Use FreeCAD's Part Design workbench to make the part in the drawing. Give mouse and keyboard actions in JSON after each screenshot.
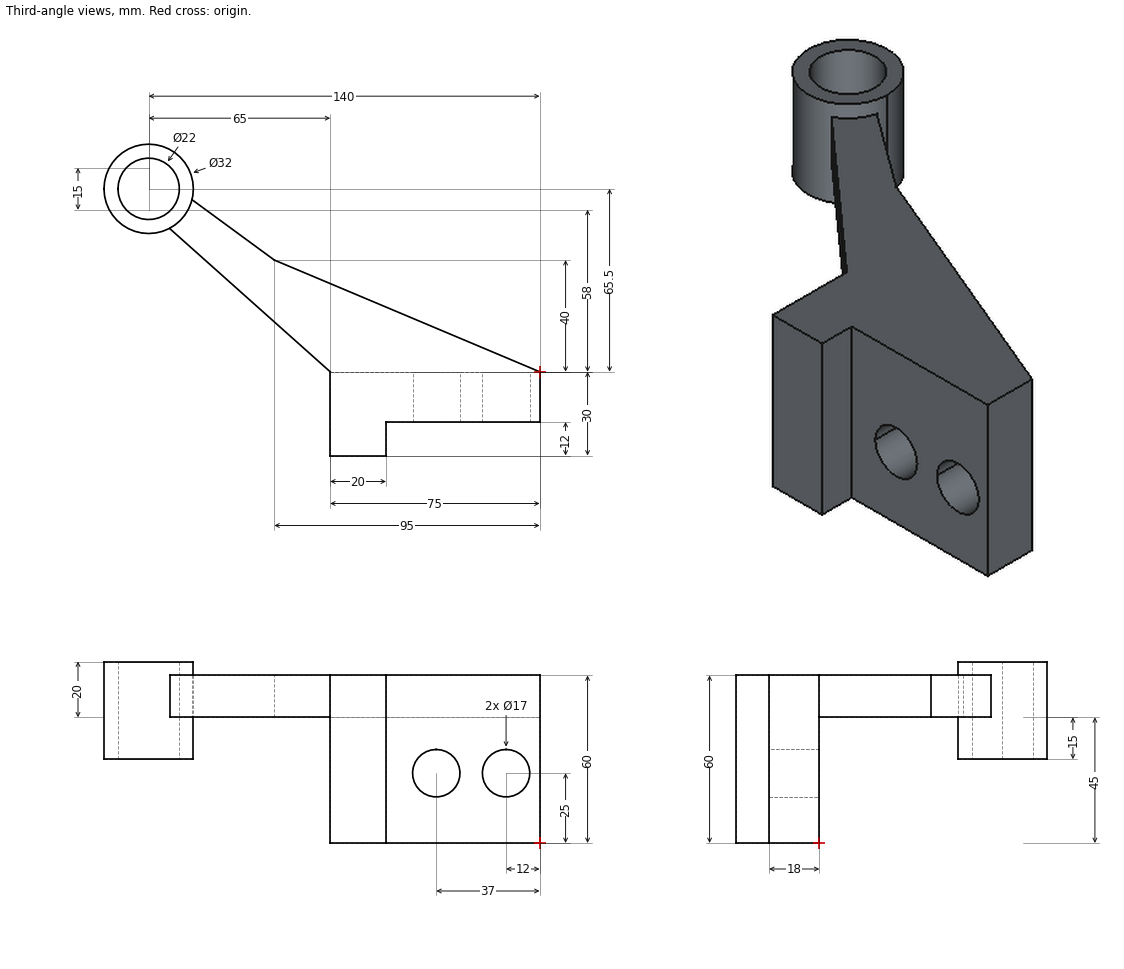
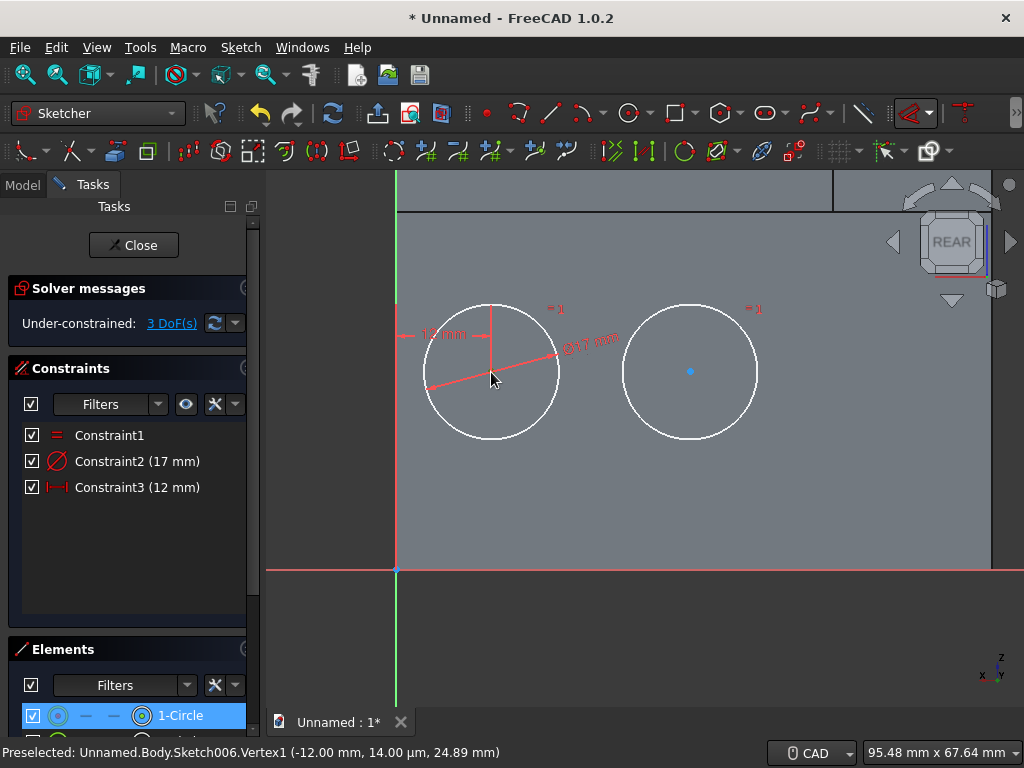
{"action": "left_click", "coordinate": [932, 114]}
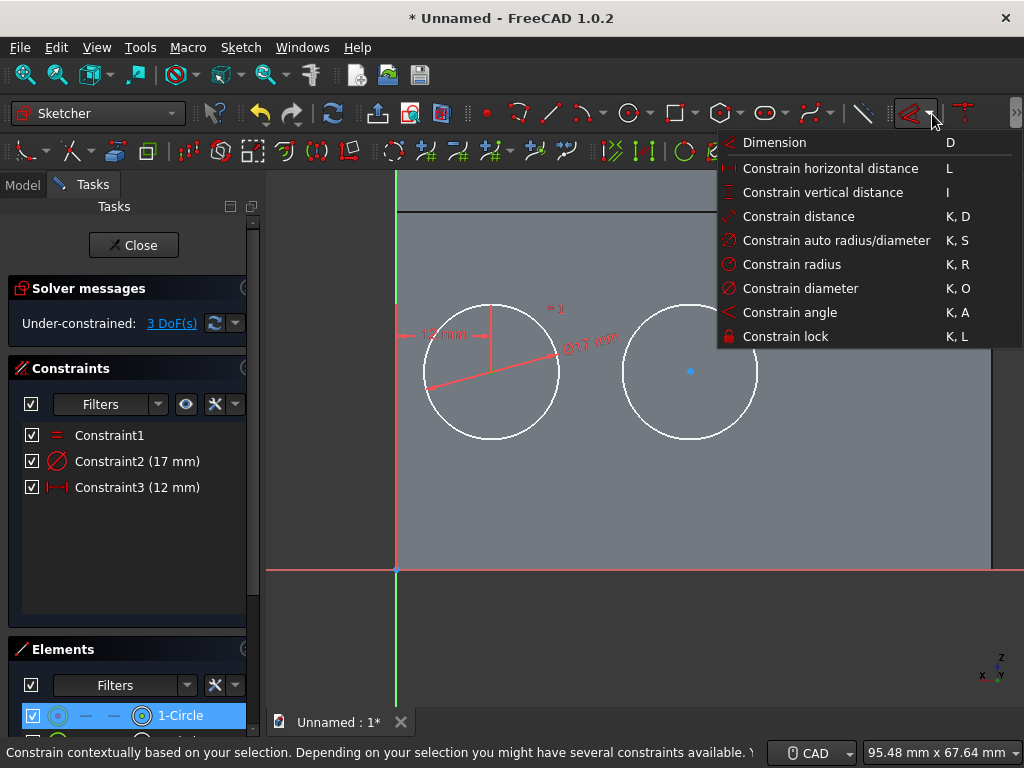
{"action": "left_click", "coordinate": [870, 192]}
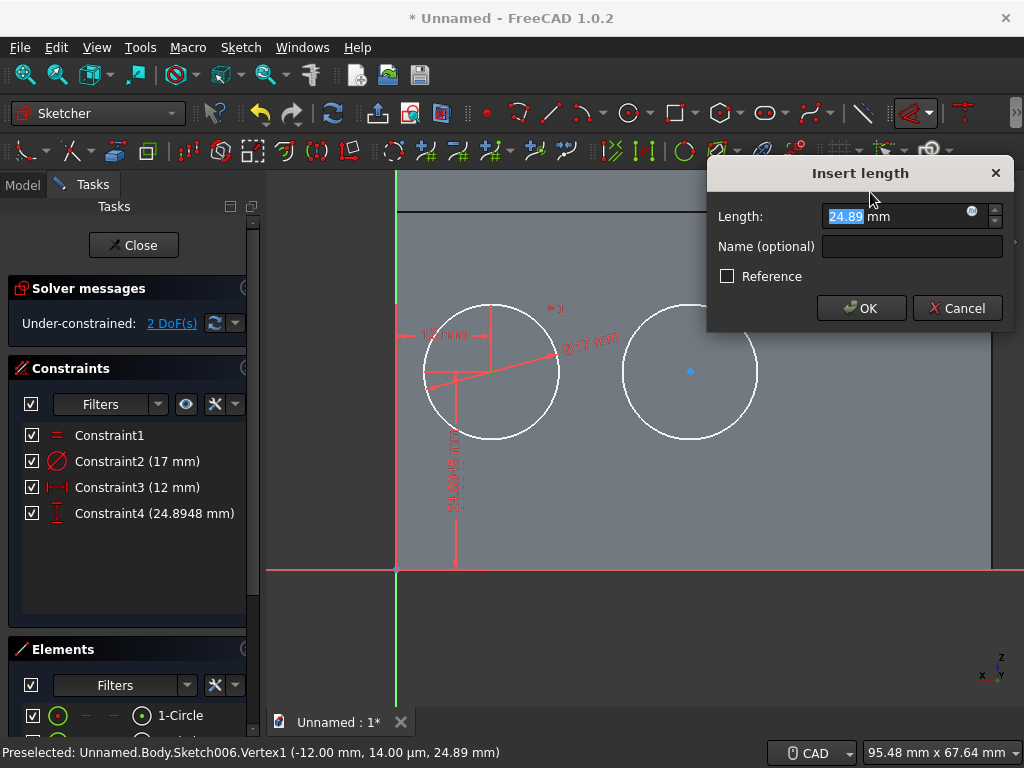
{"action": "type", "text": "25"}
{"action": "key", "text": "Return"}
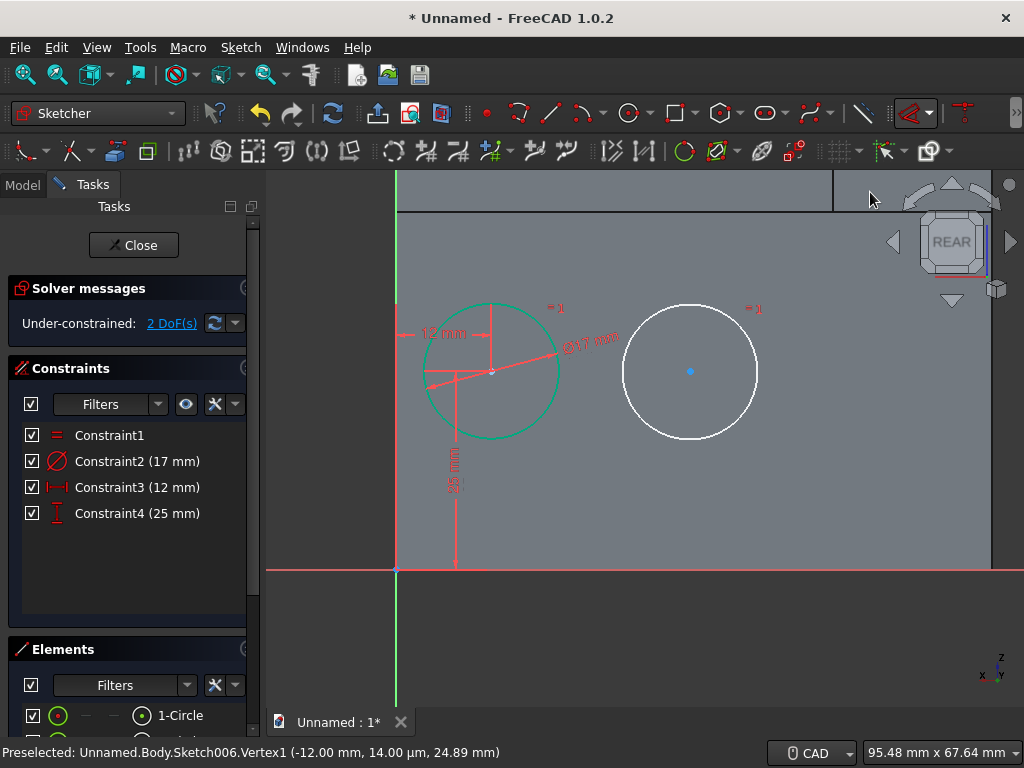
{"action": "left_click", "coordinate": [690, 372]}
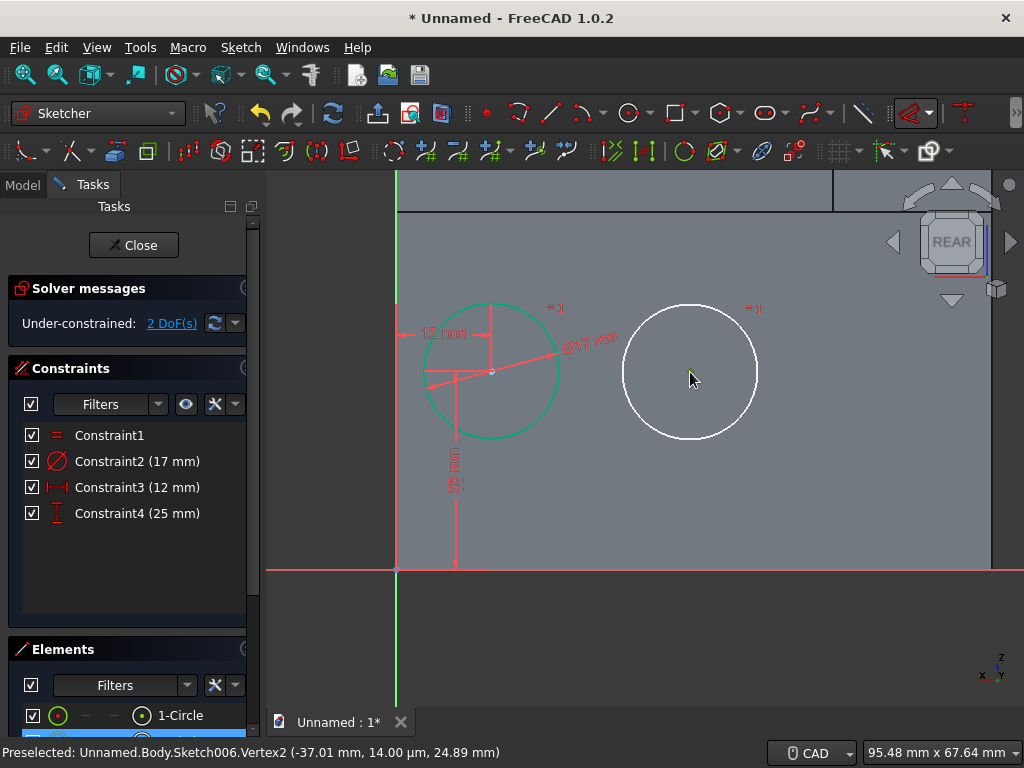
{"action": "left_click", "coordinate": [932, 114]}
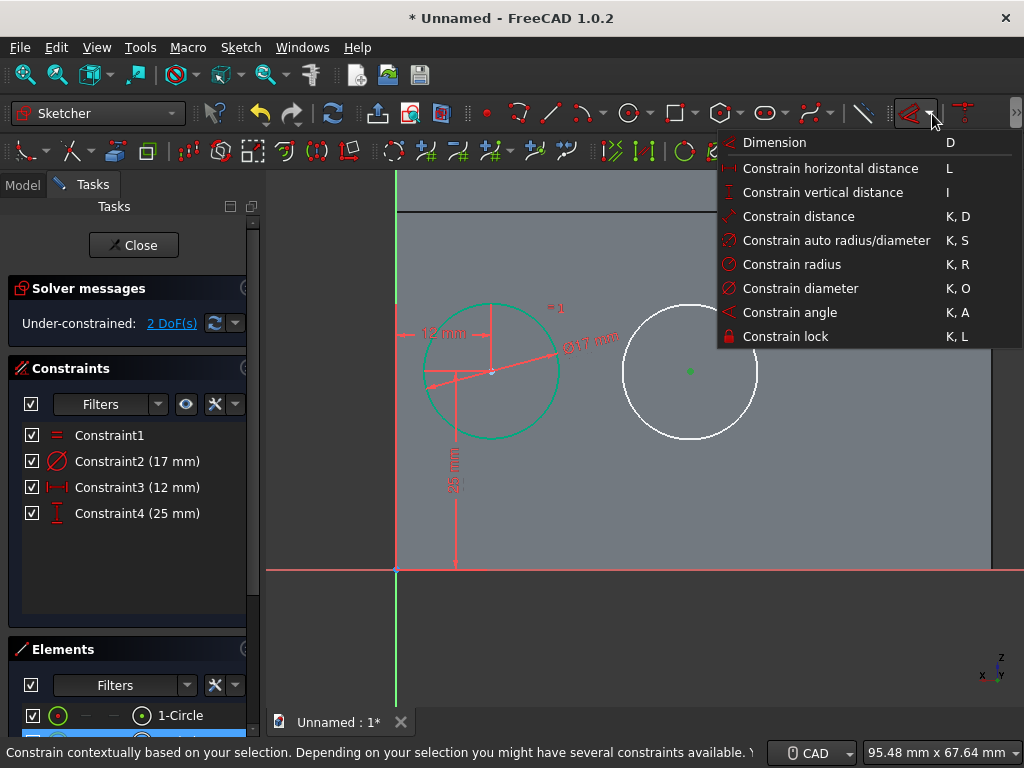
{"action": "left_click", "coordinate": [870, 168]}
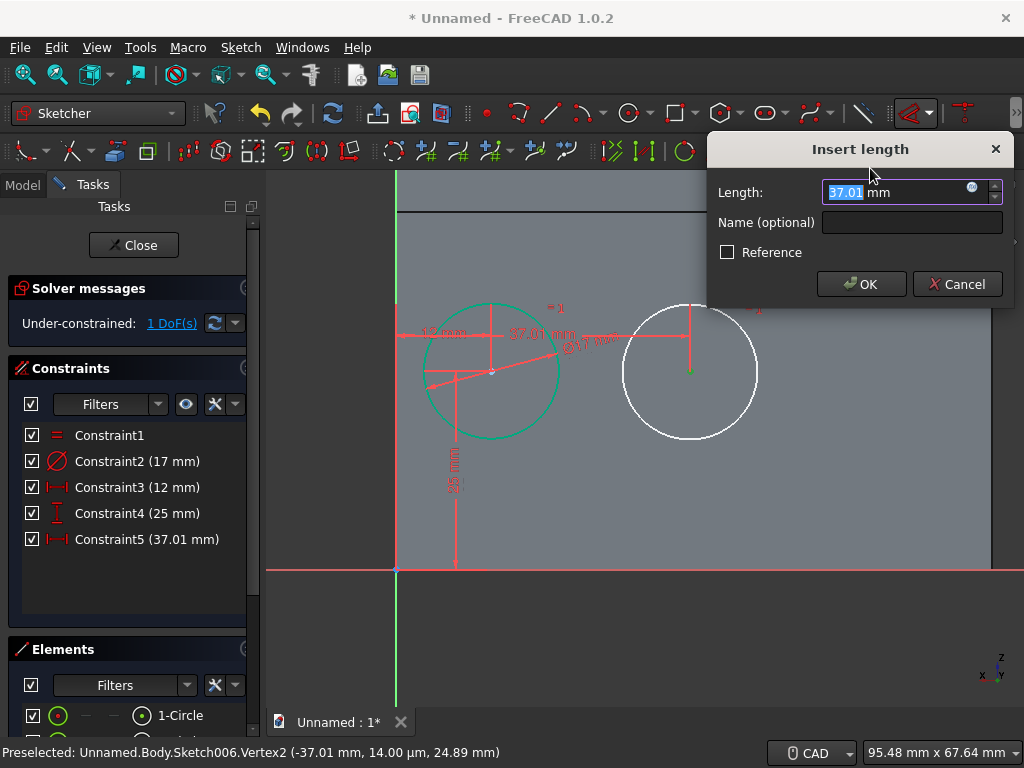
{"action": "type", "text": "37"}
{"action": "key", "text": "Return"}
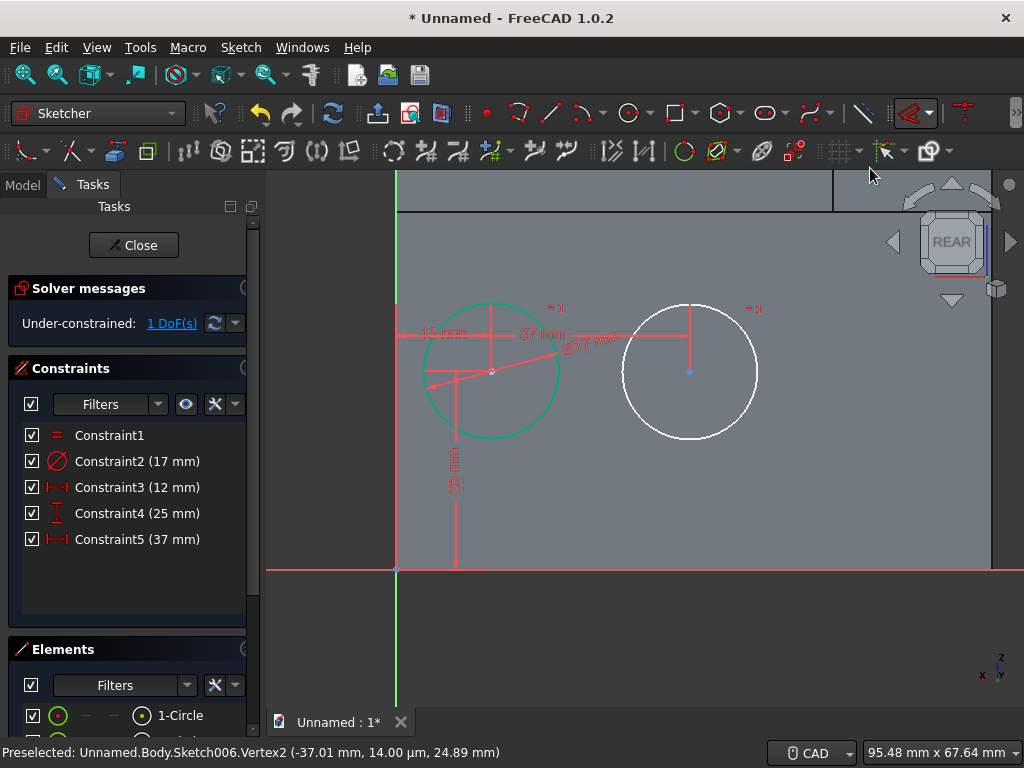
{"action": "left_click", "coordinate": [690, 372]}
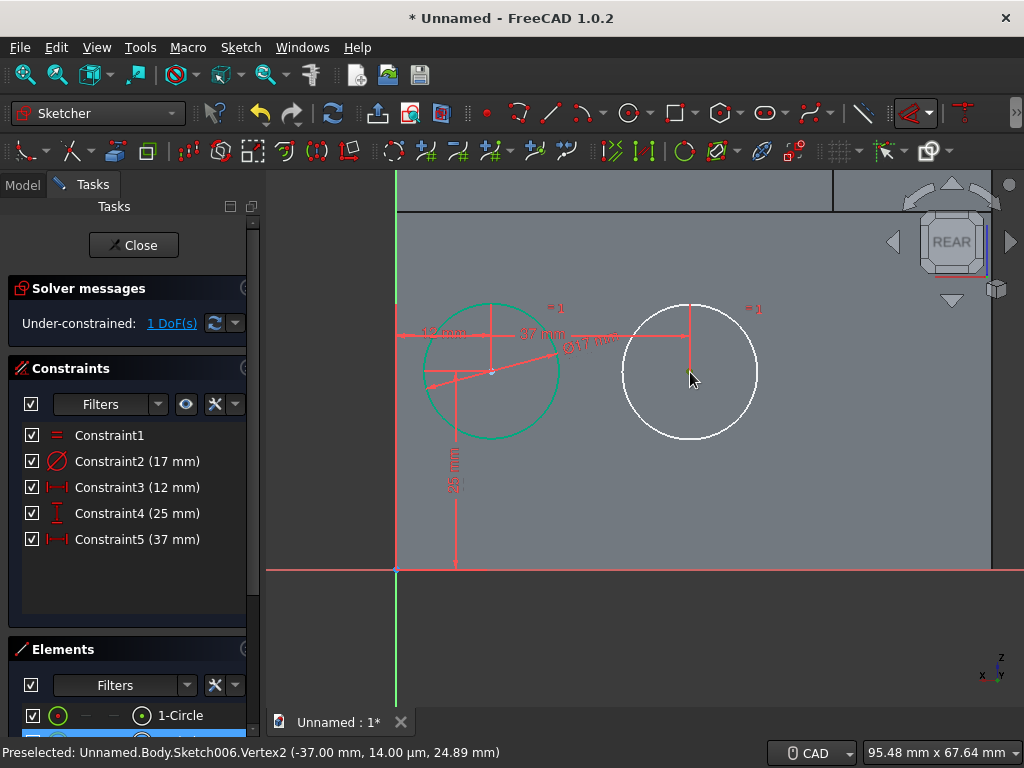
{"action": "left_click", "coordinate": [932, 114]}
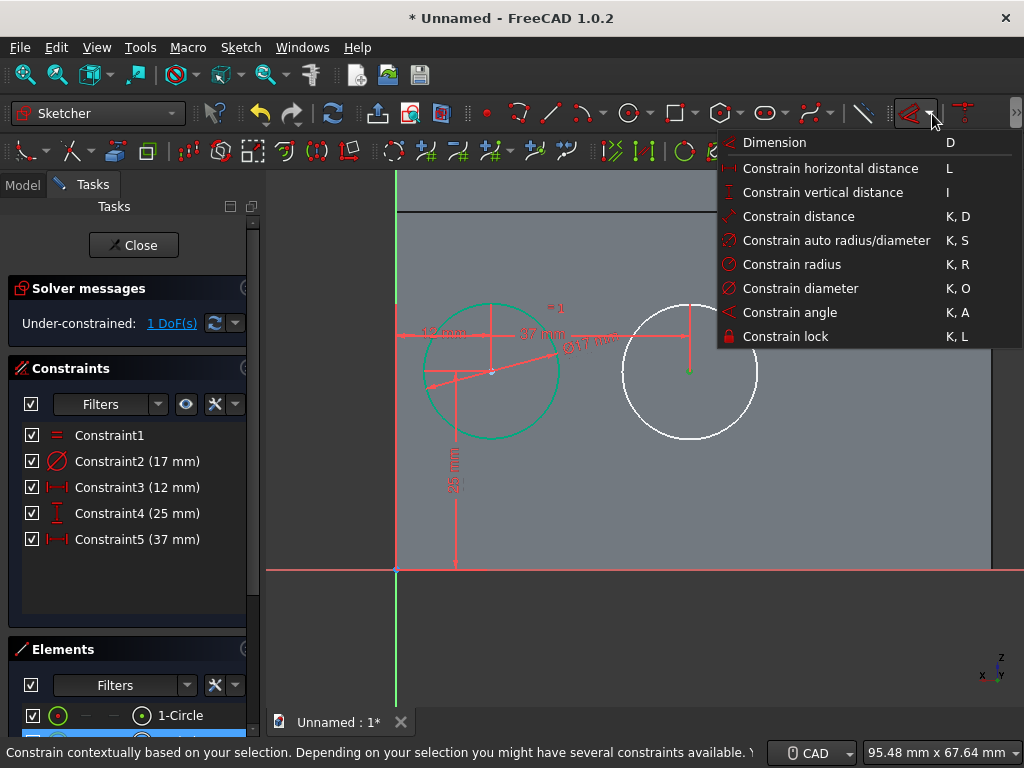
{"action": "left_click", "coordinate": [870, 192]}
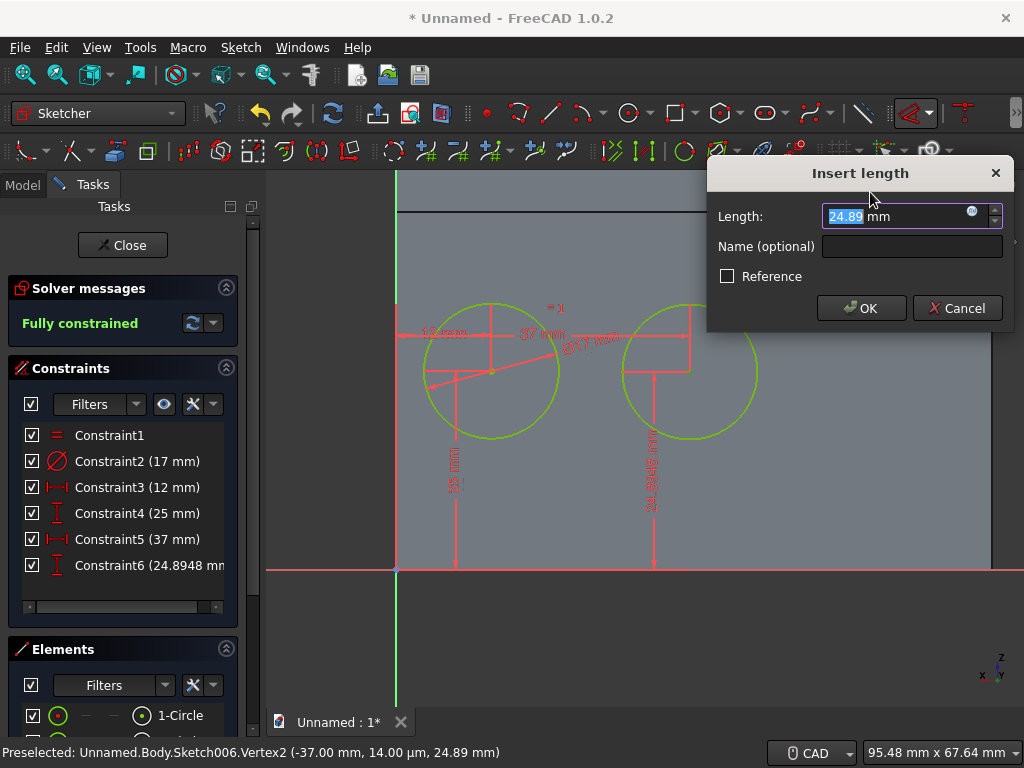
{"action": "type", "text": "25"}
{"action": "key", "text": "Return"}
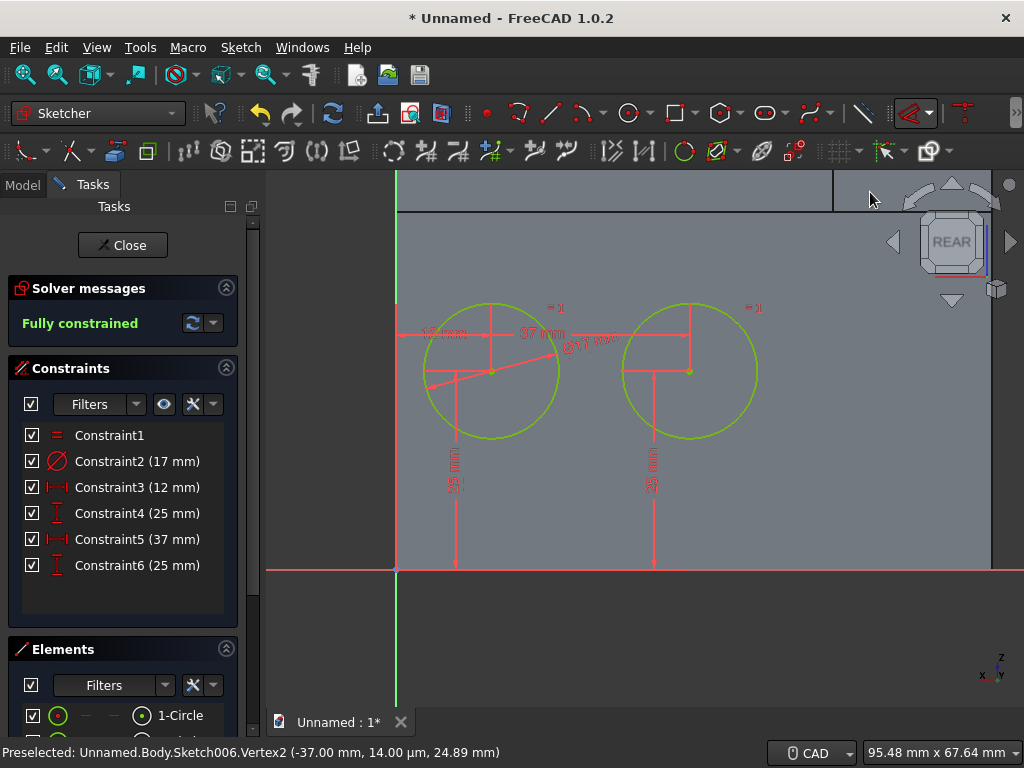
{"action": "left_click", "coordinate": [123, 245]}